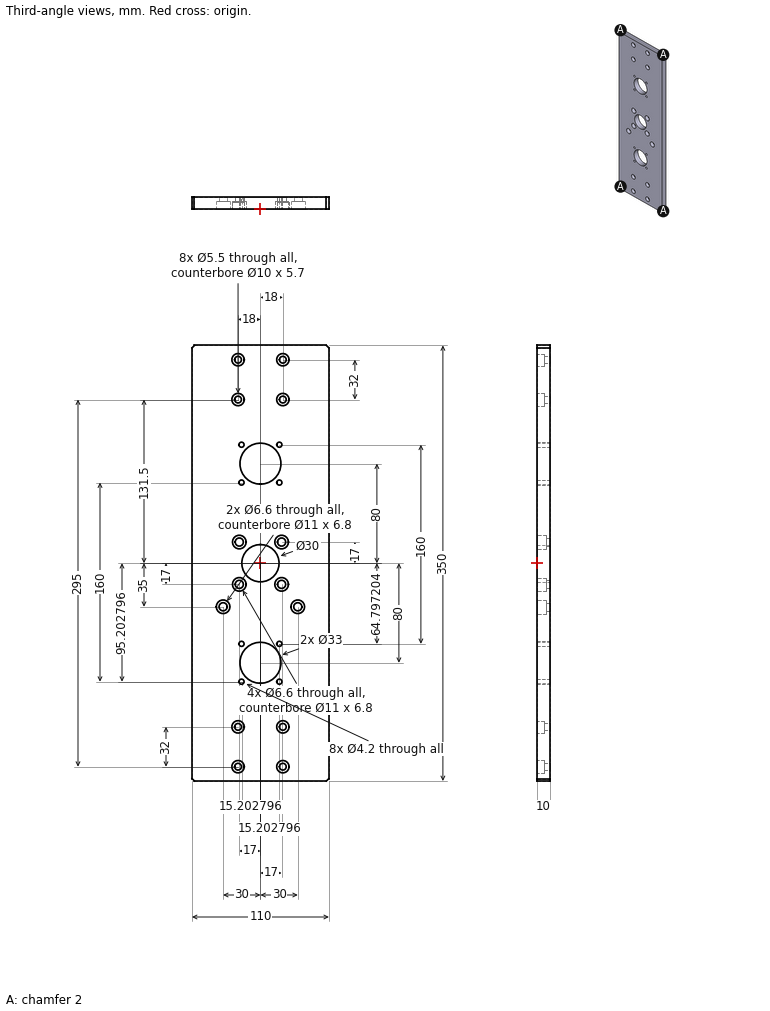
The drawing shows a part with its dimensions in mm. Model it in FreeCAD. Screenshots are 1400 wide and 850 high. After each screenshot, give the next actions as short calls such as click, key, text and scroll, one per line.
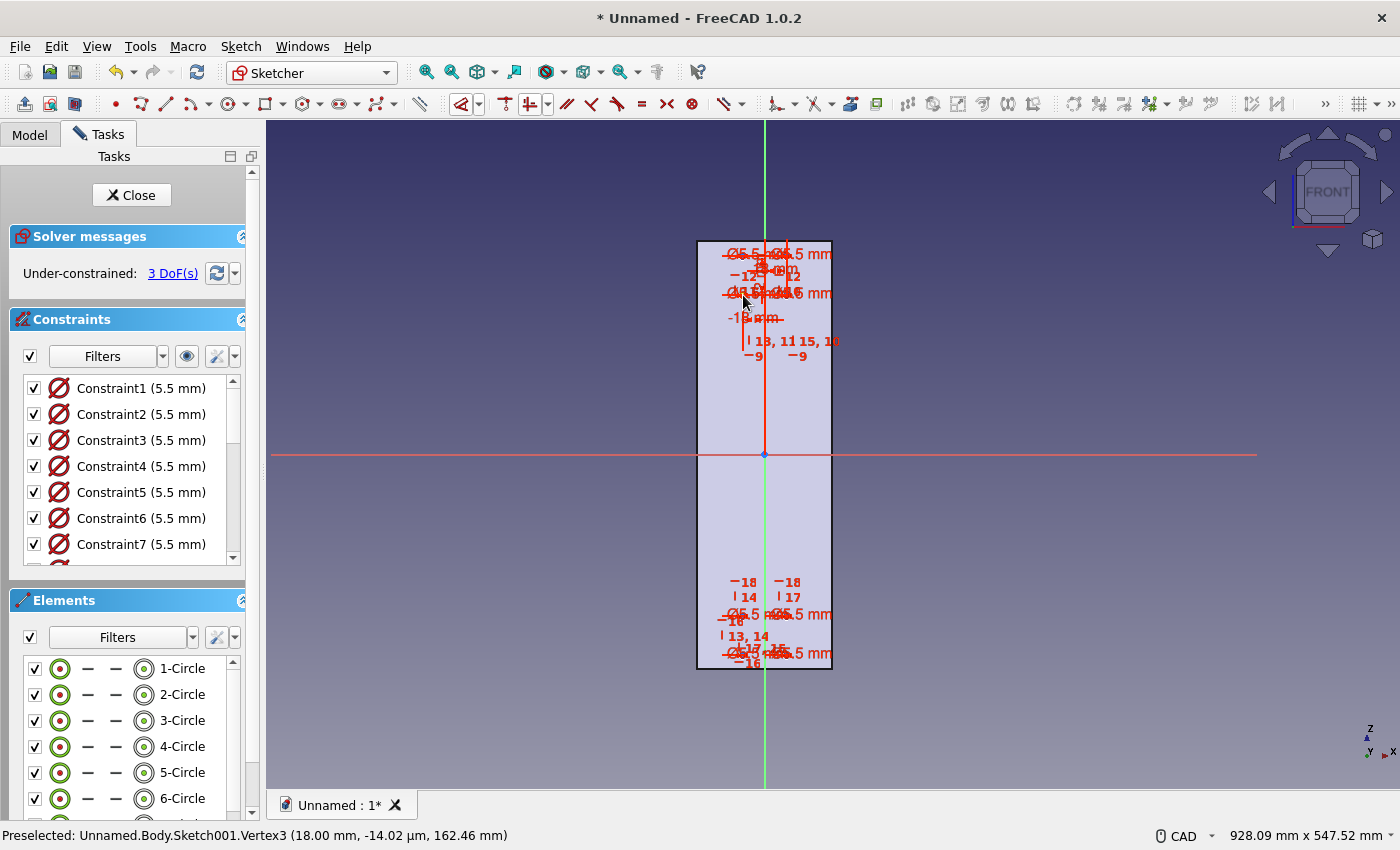
click(743, 655)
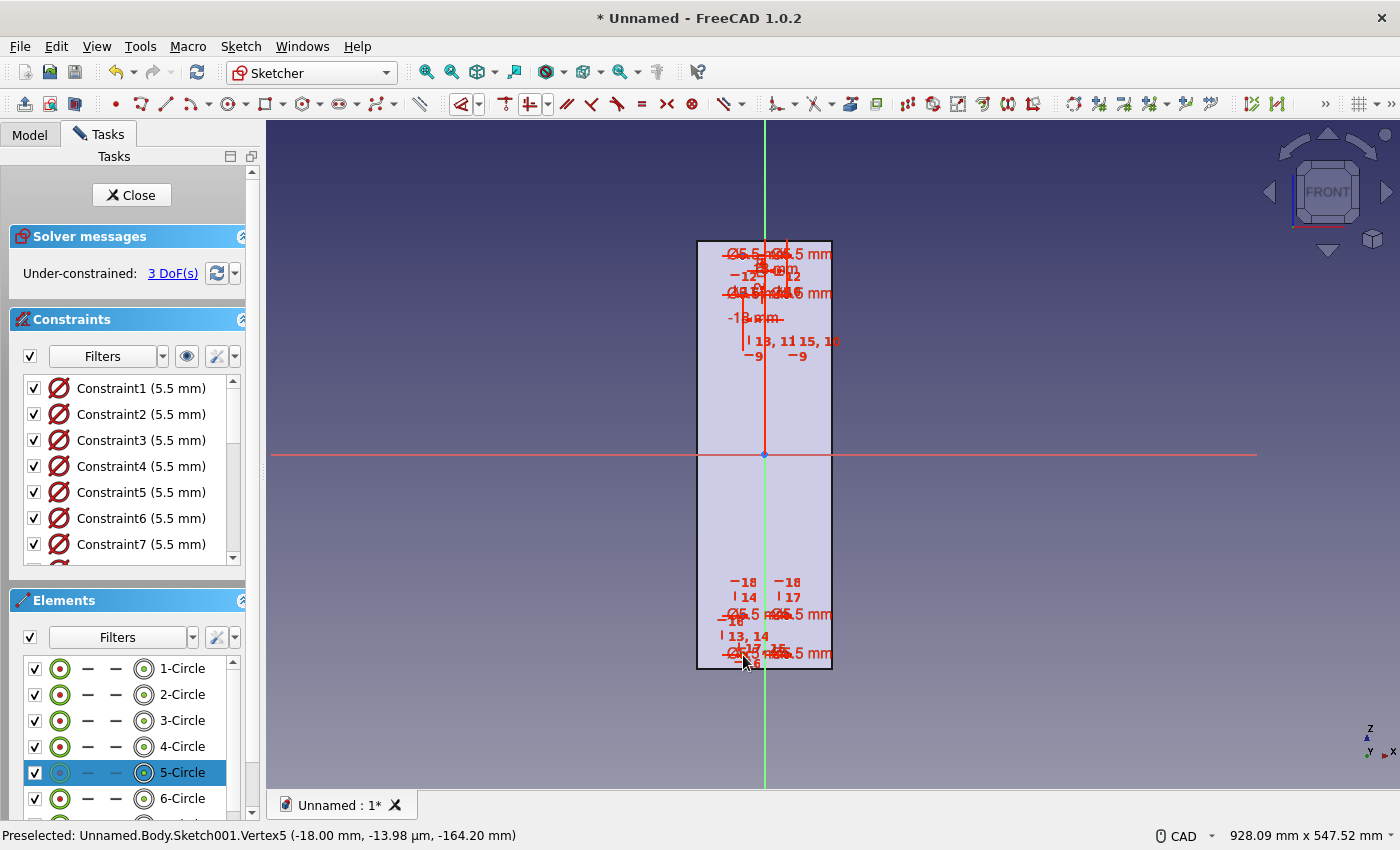
click(743, 616)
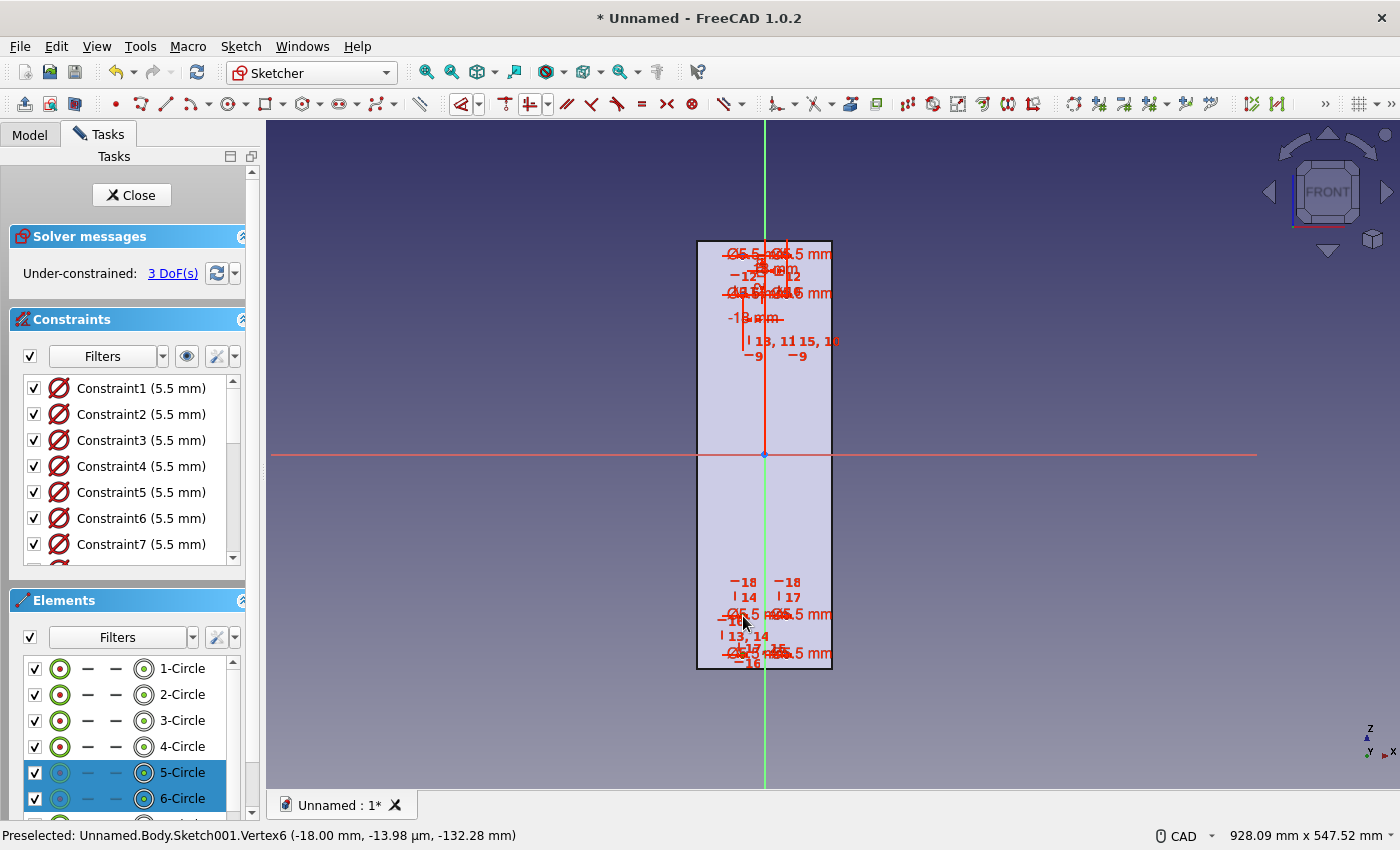
key(i)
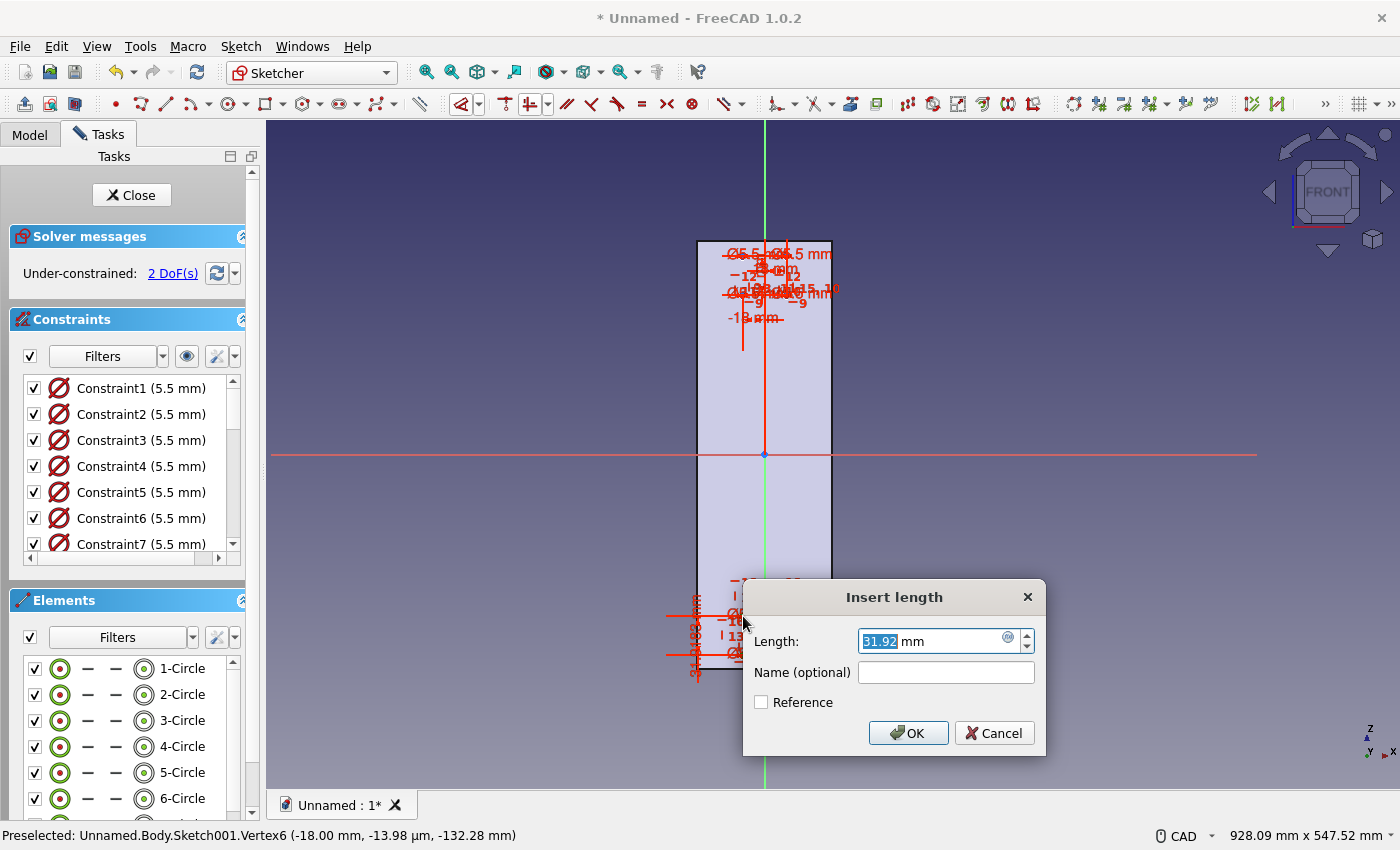
text(32)
key(Return)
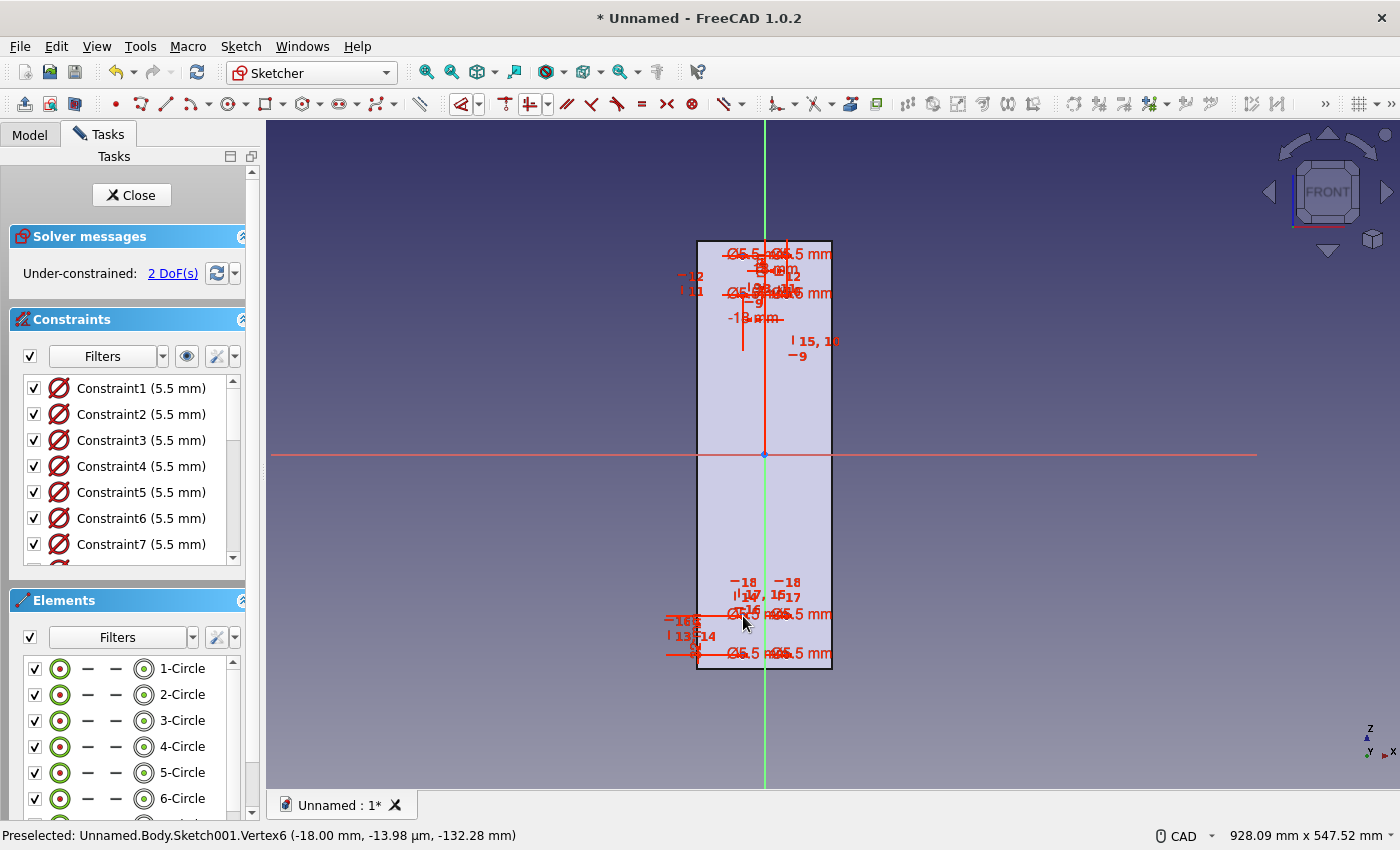
click(743, 295)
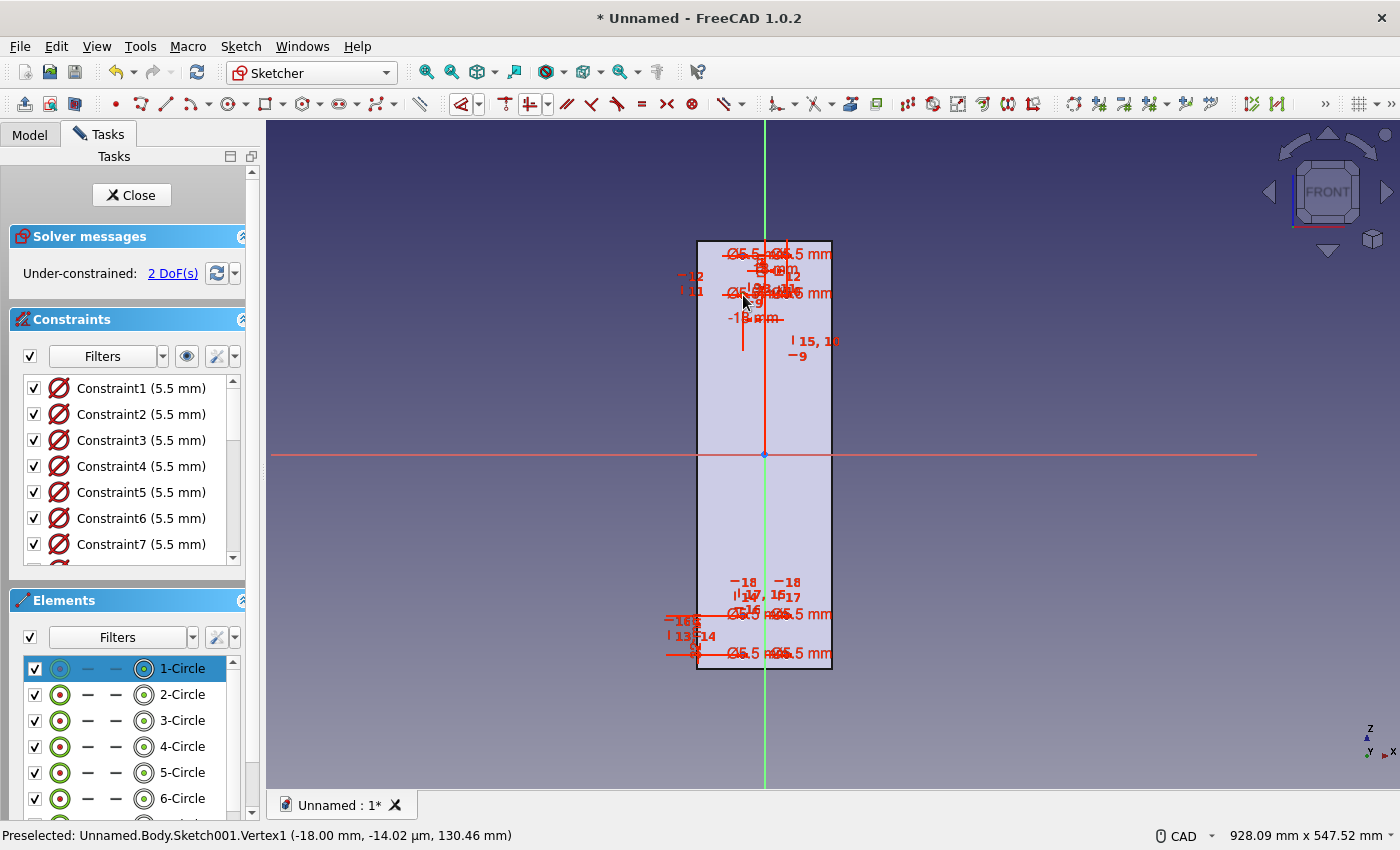
click(743, 655)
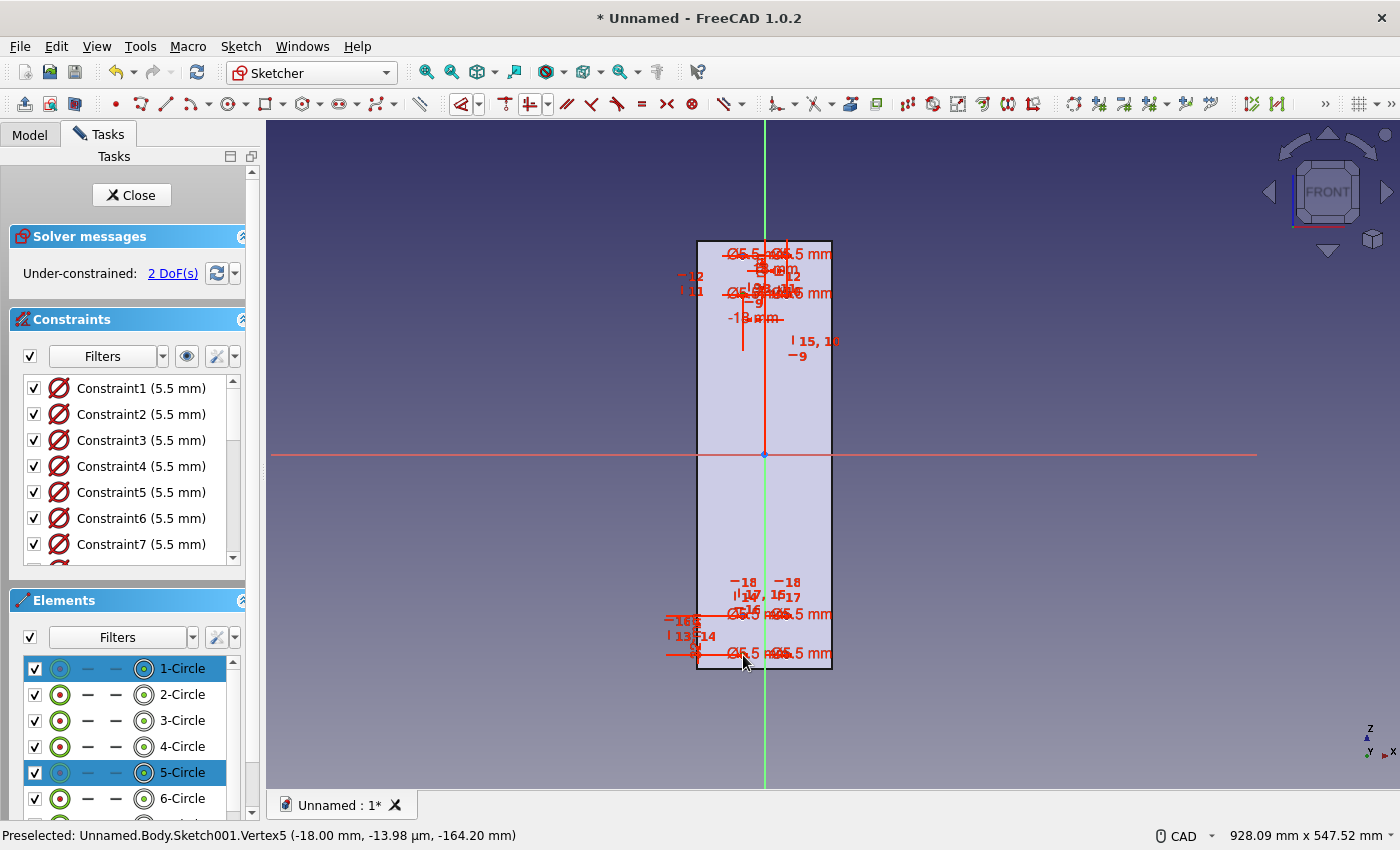
key(i)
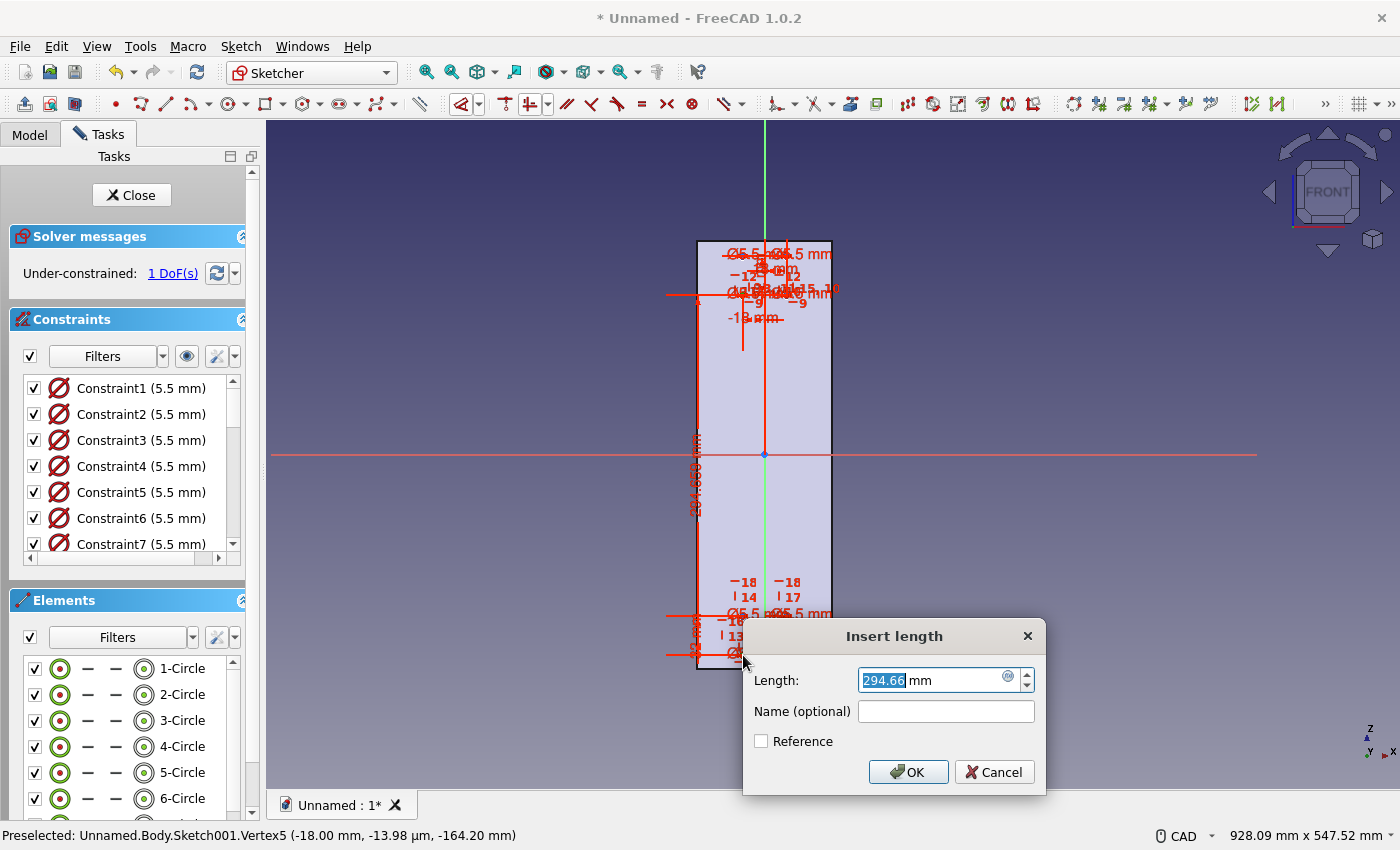
text(295)
key(Return)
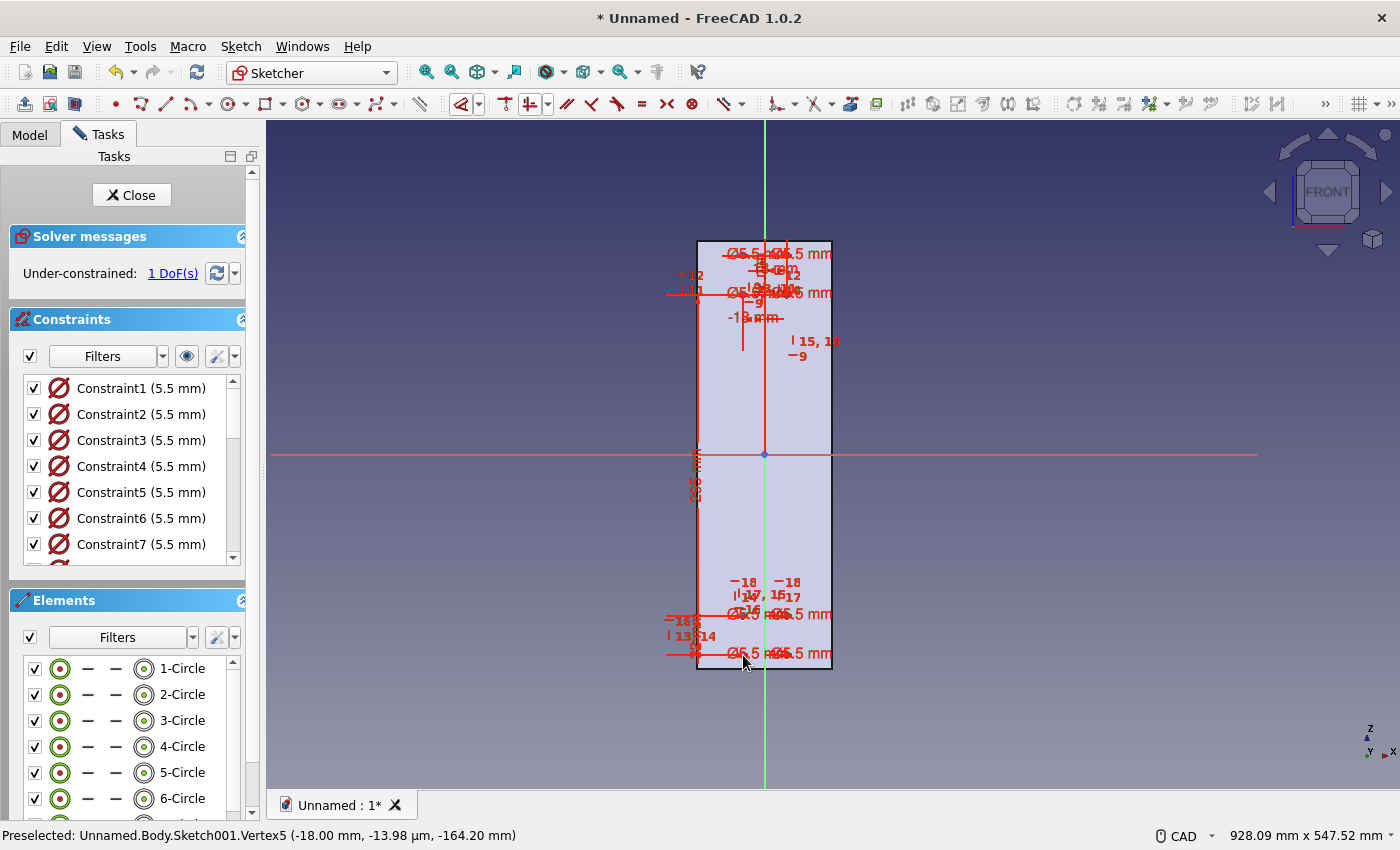
click(743, 295)